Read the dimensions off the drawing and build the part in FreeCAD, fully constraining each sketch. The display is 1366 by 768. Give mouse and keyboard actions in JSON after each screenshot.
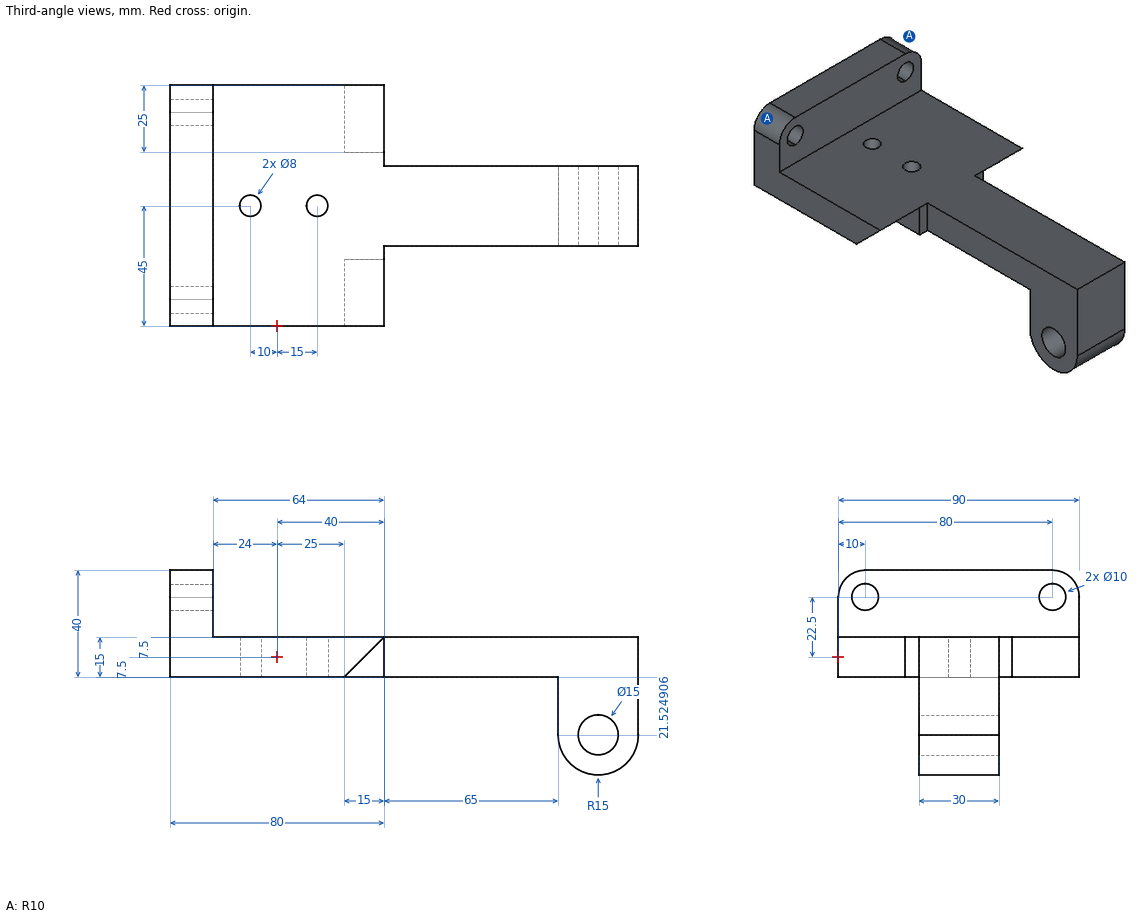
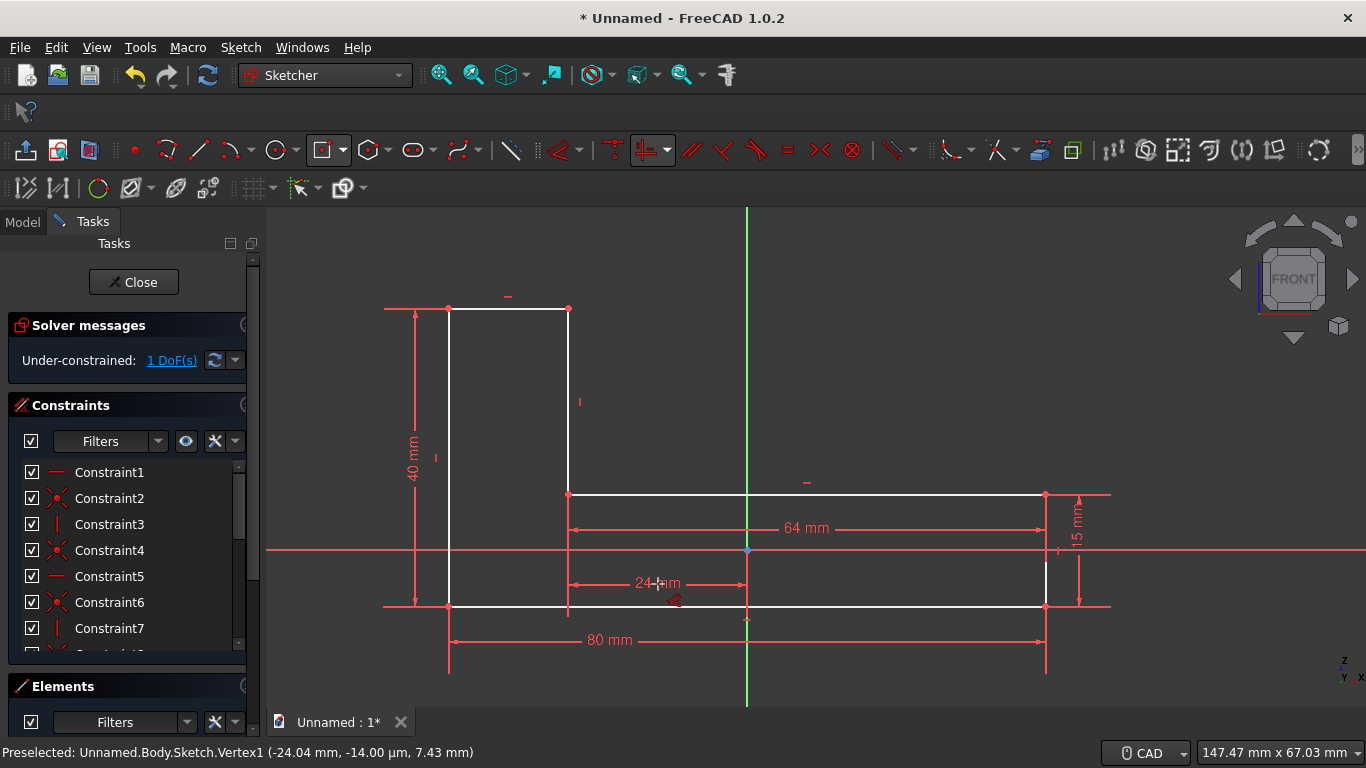
{"action": "left_click", "coordinate": [568, 495]}
{"action": "left_click", "coordinate": [534, 523]}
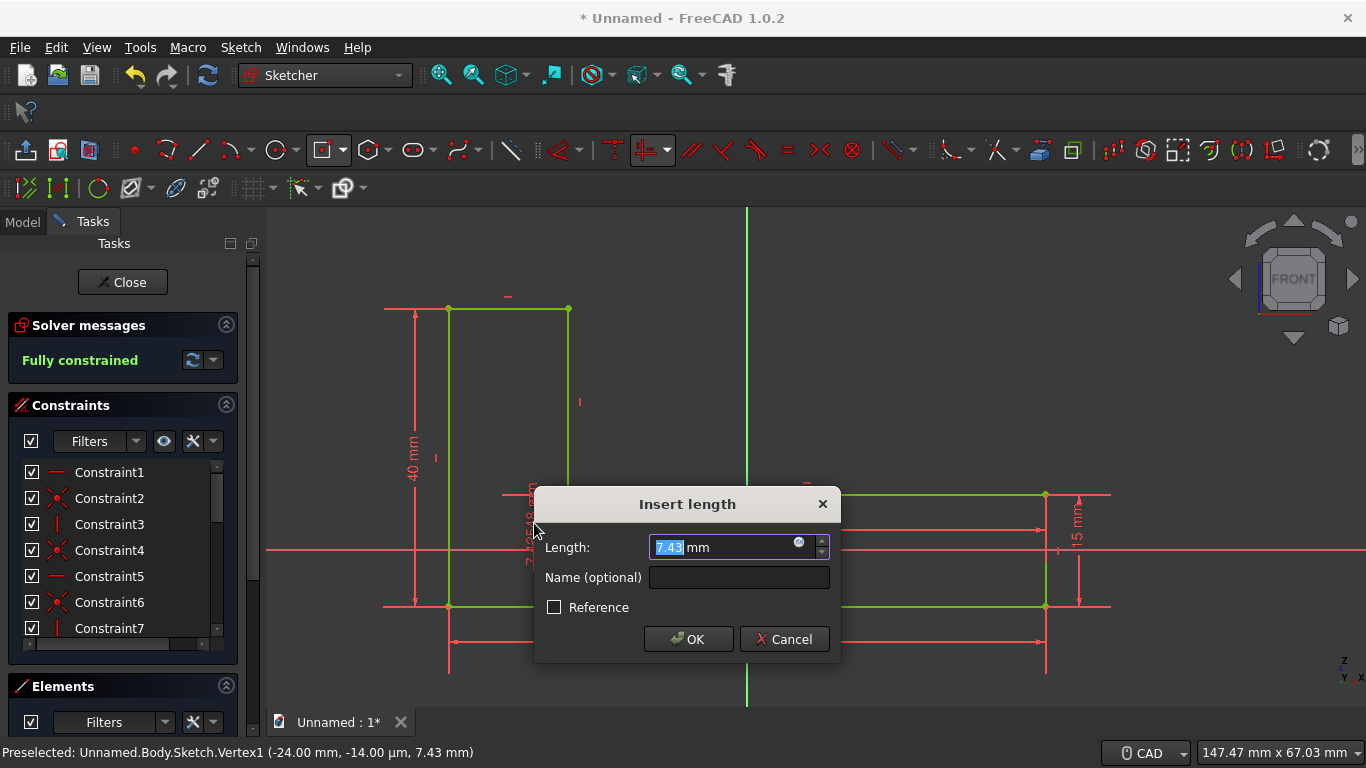
{"action": "type", "text": "7.5"}
{"action": "key", "text": "Return"}
{"action": "key", "text": "Escape"}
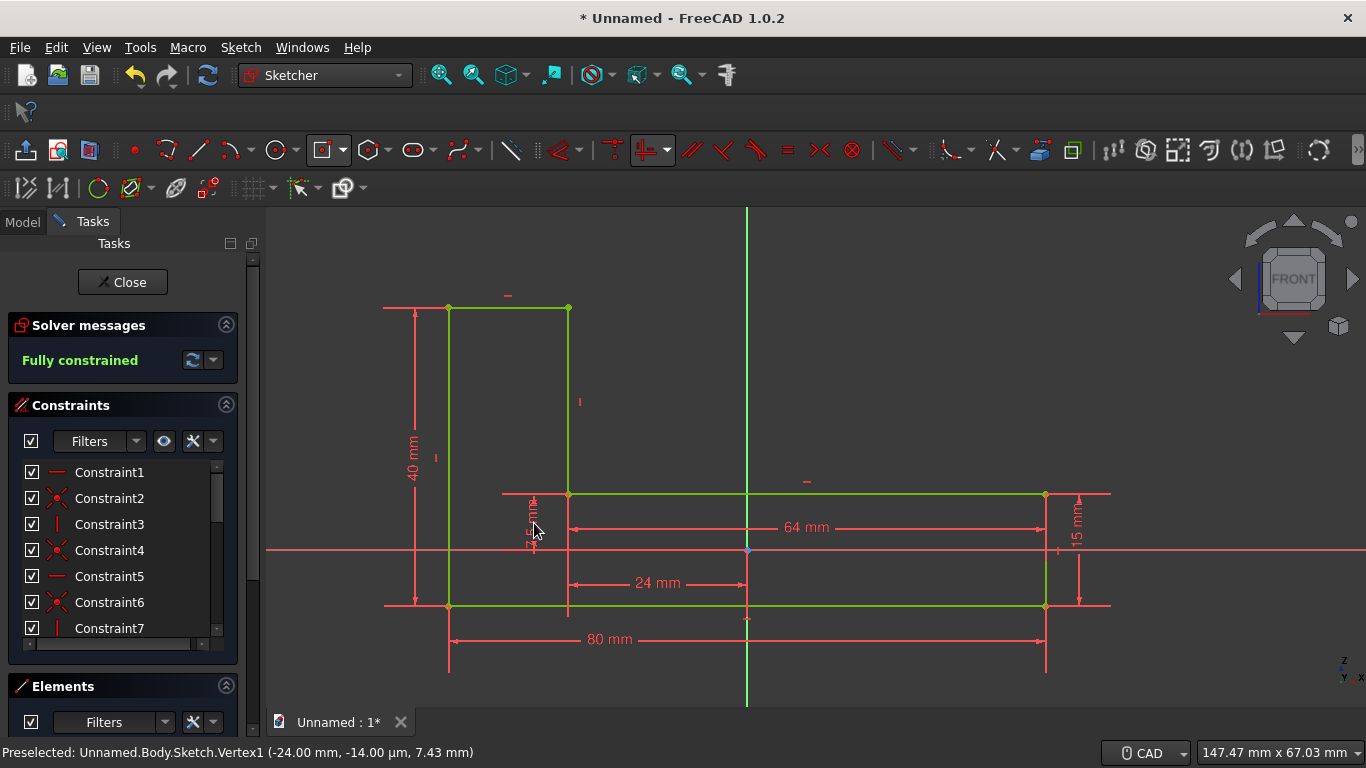
{"action": "left_click", "coordinate": [123, 282]}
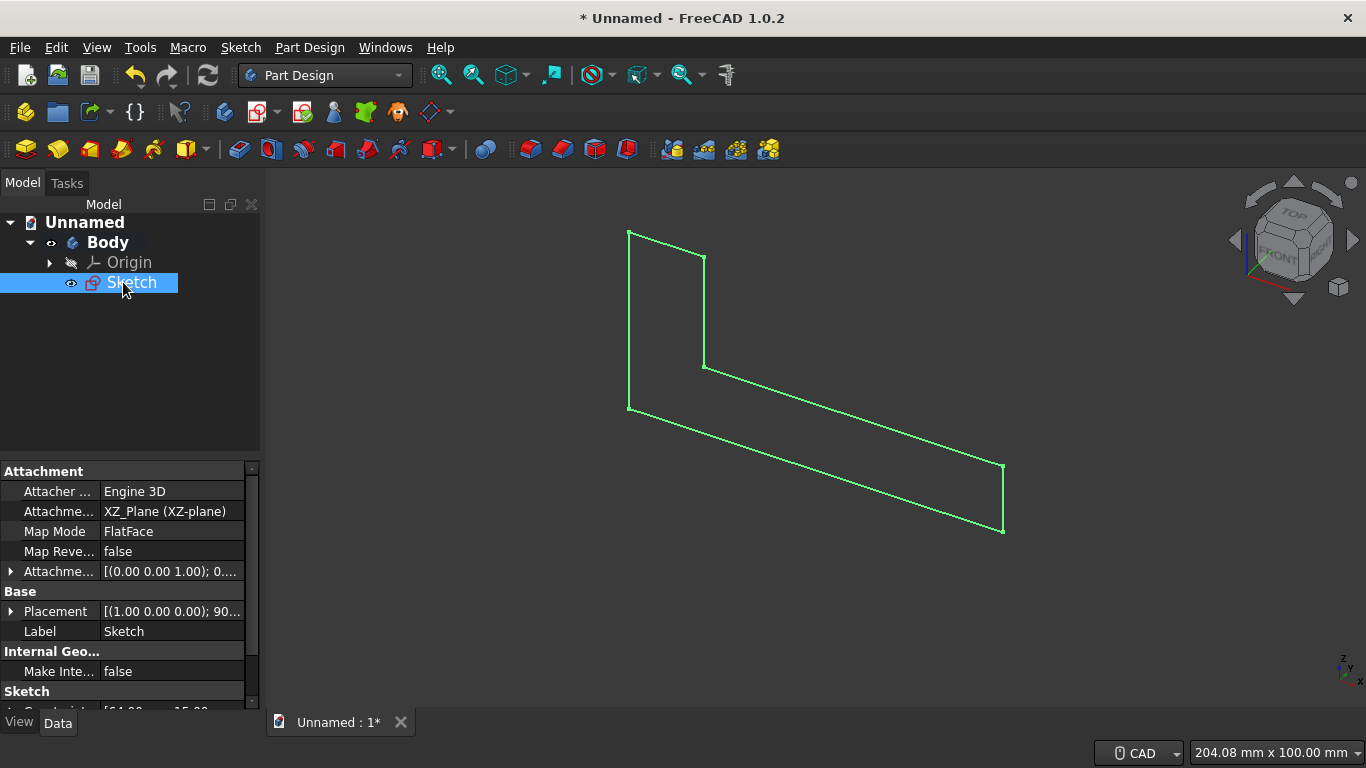
{"action": "left_click", "coordinate": [26, 150]}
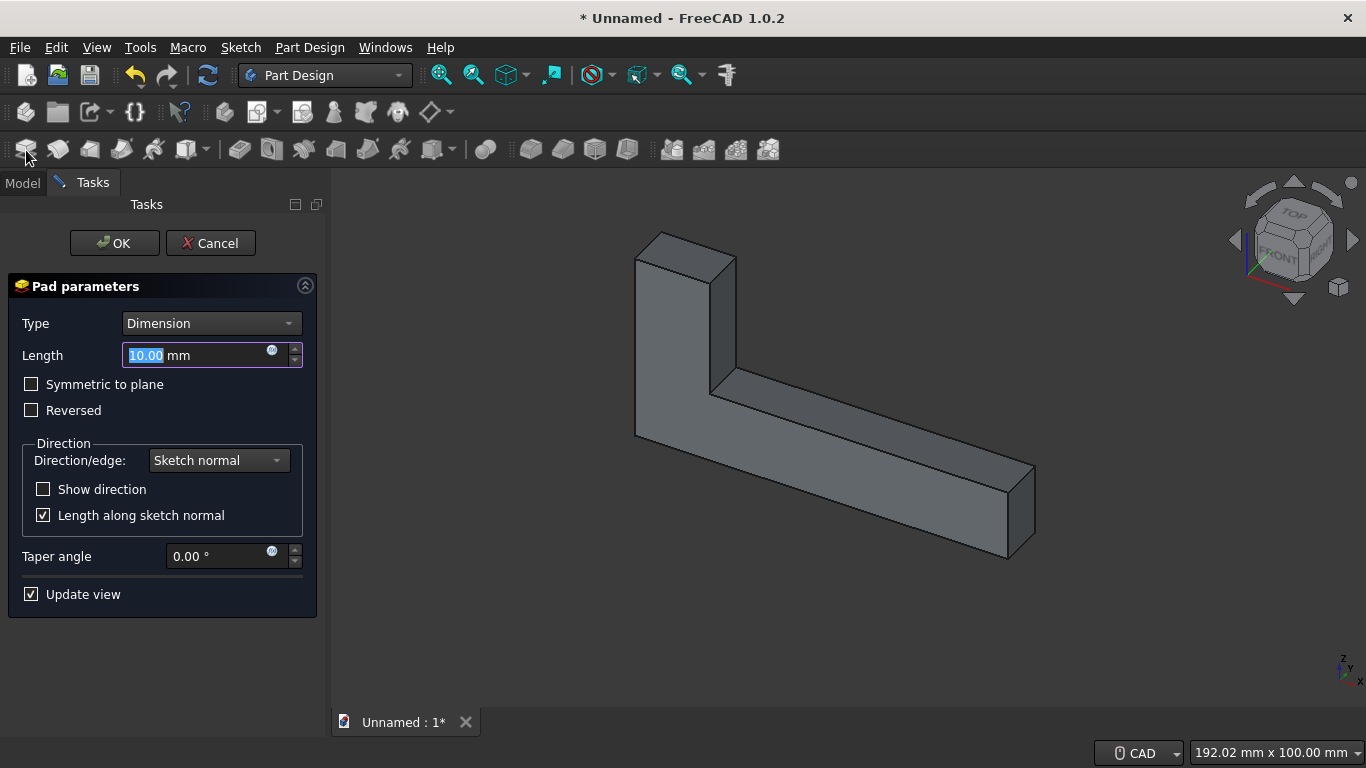
{"action": "type", "text": "90"}
{"action": "key", "text": "Tab"}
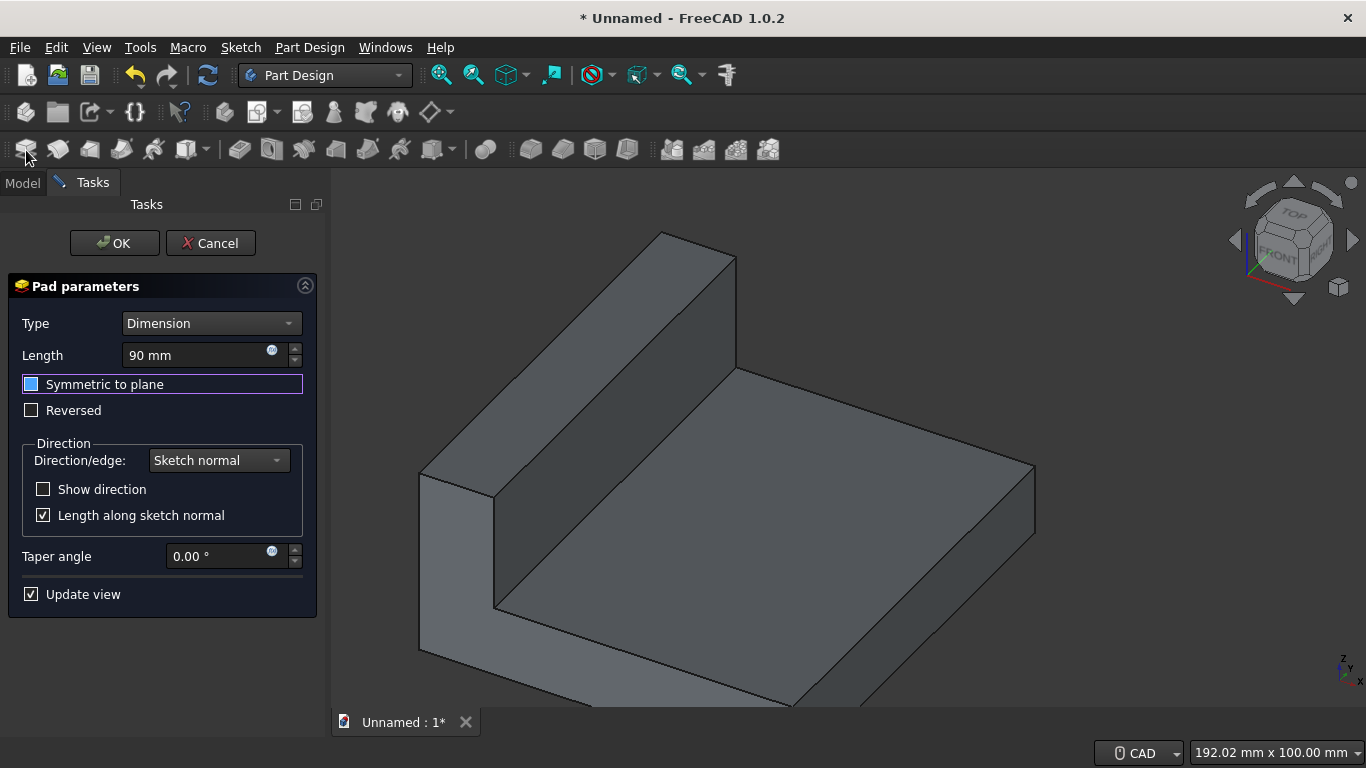
{"action": "left_click", "coordinate": [30, 410]}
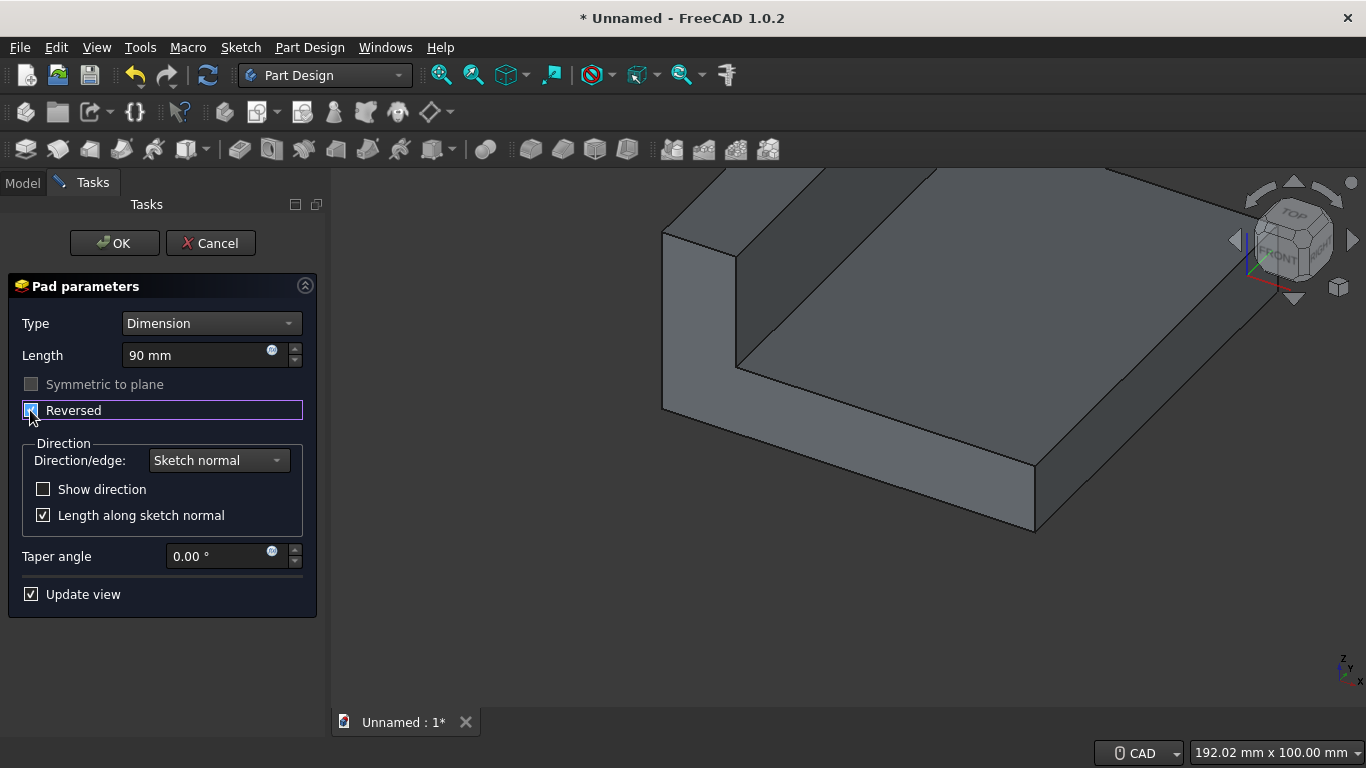
{"action": "left_click", "coordinate": [115, 243]}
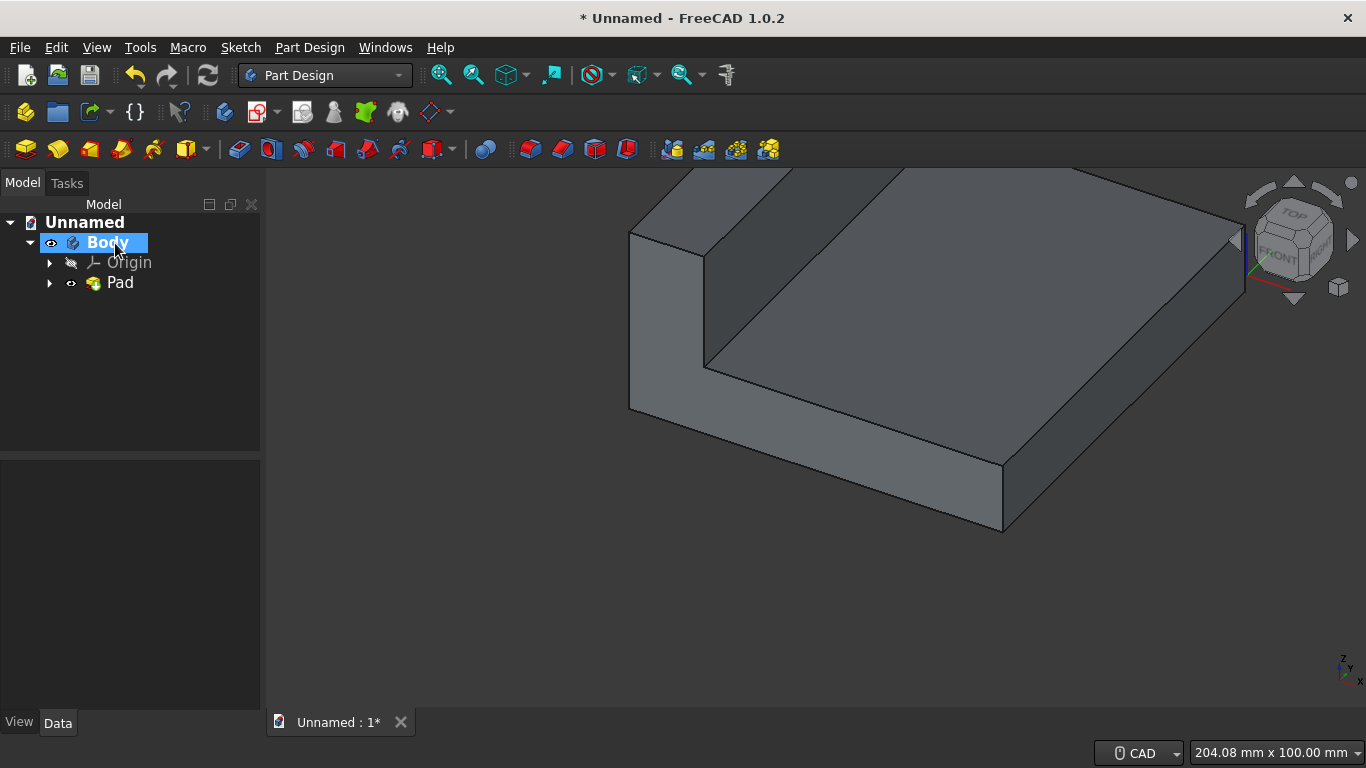
{"action": "left_click", "coordinate": [442, 76]}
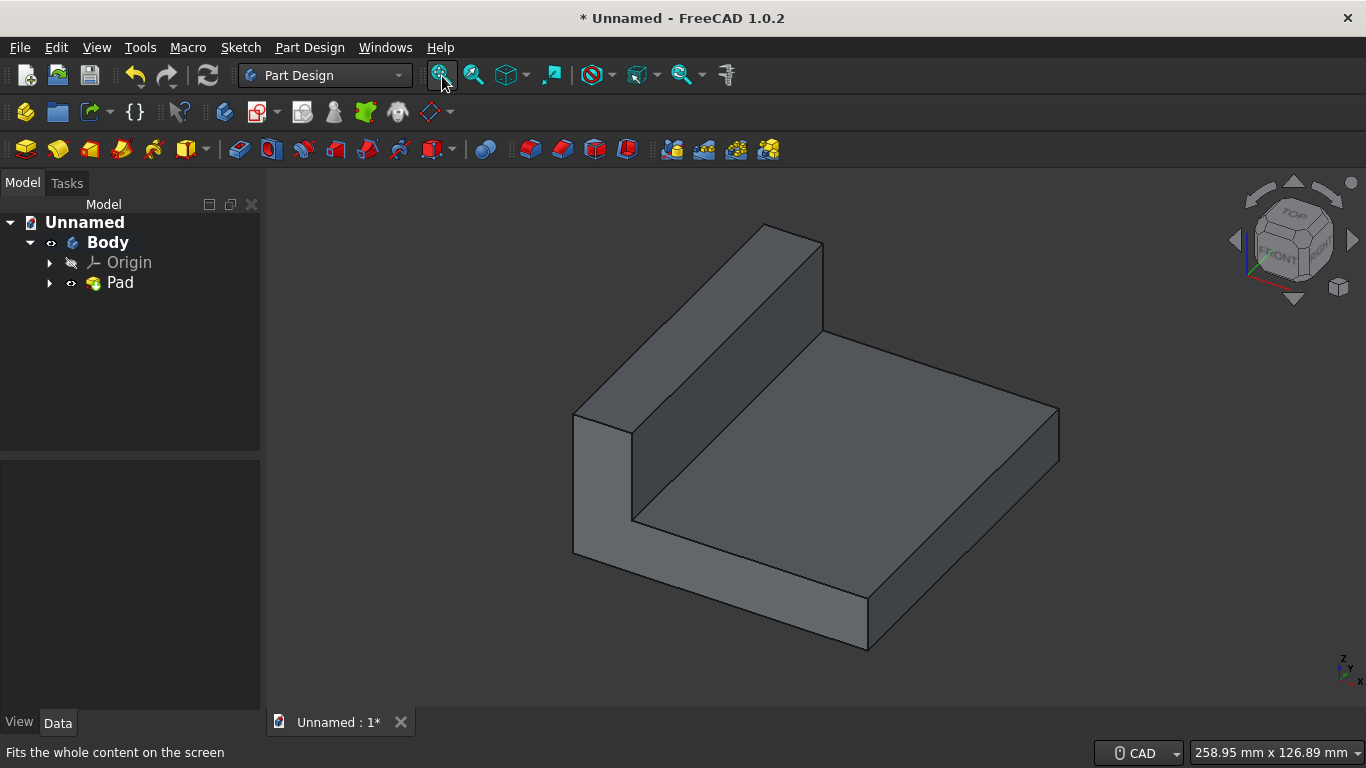
{"action": "key", "text": "4"}